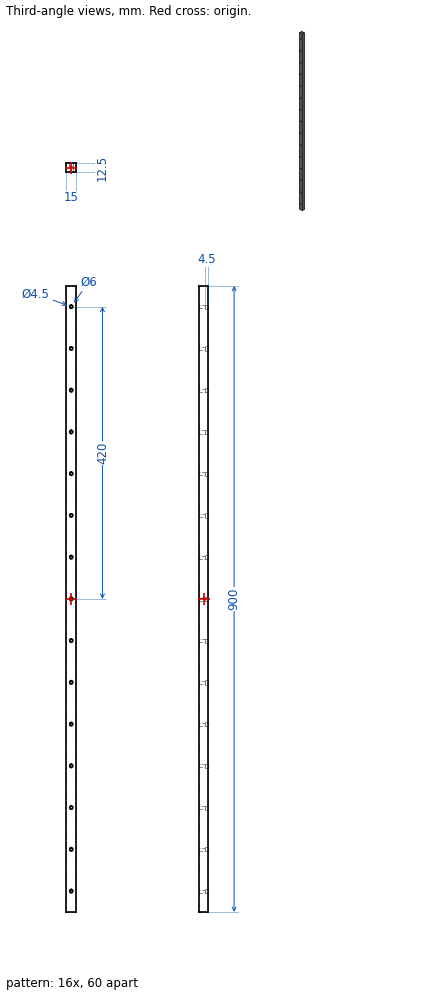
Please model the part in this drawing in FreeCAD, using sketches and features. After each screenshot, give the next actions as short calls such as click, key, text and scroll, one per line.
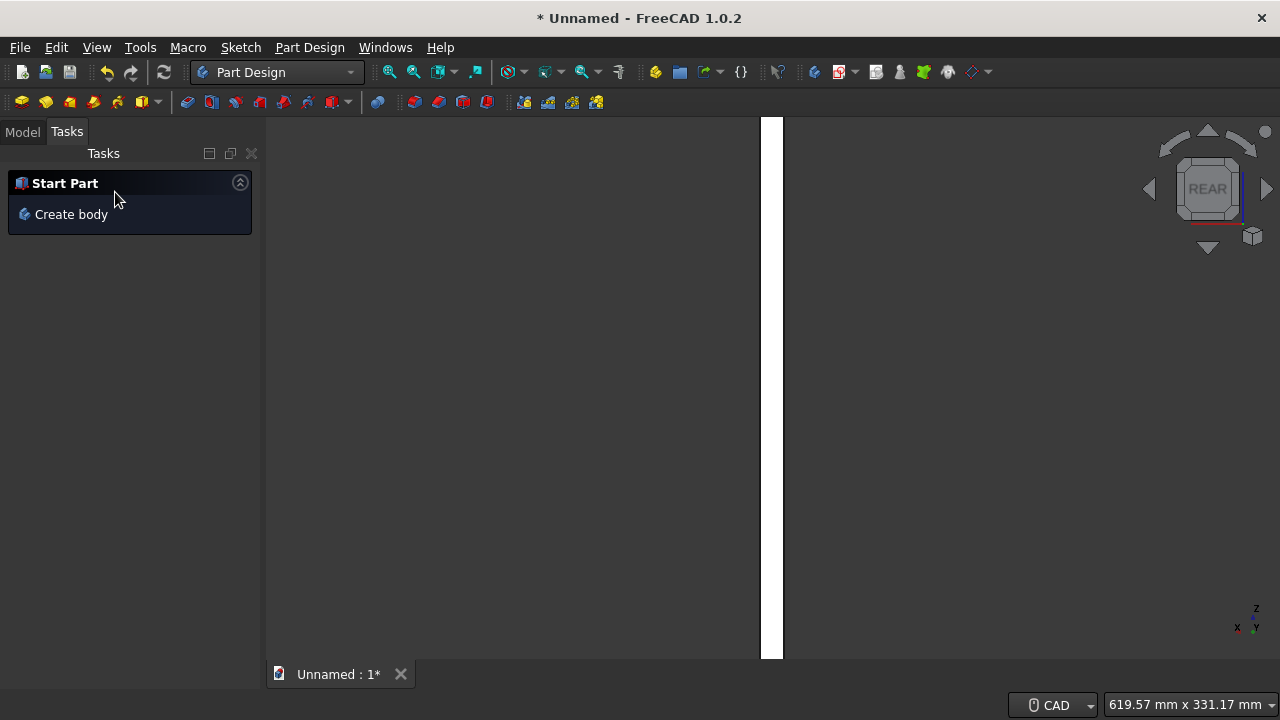
click(390, 72)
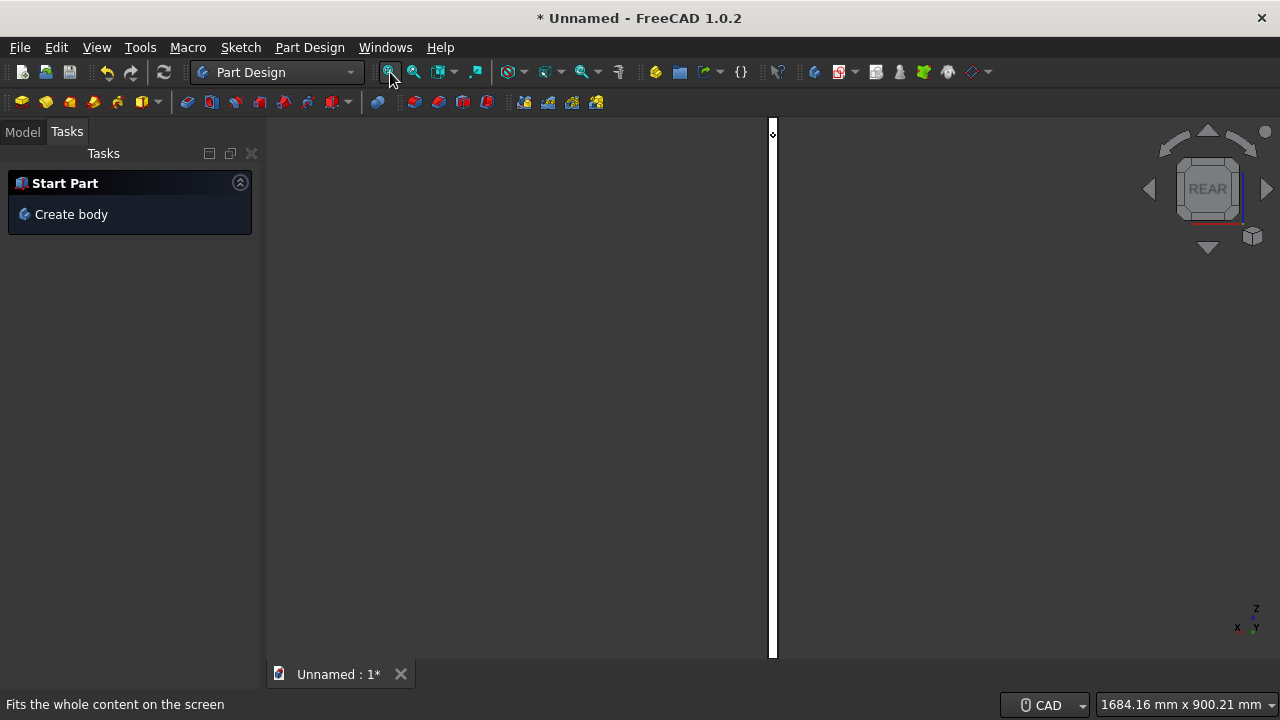
scroll(773, 155, up, 5)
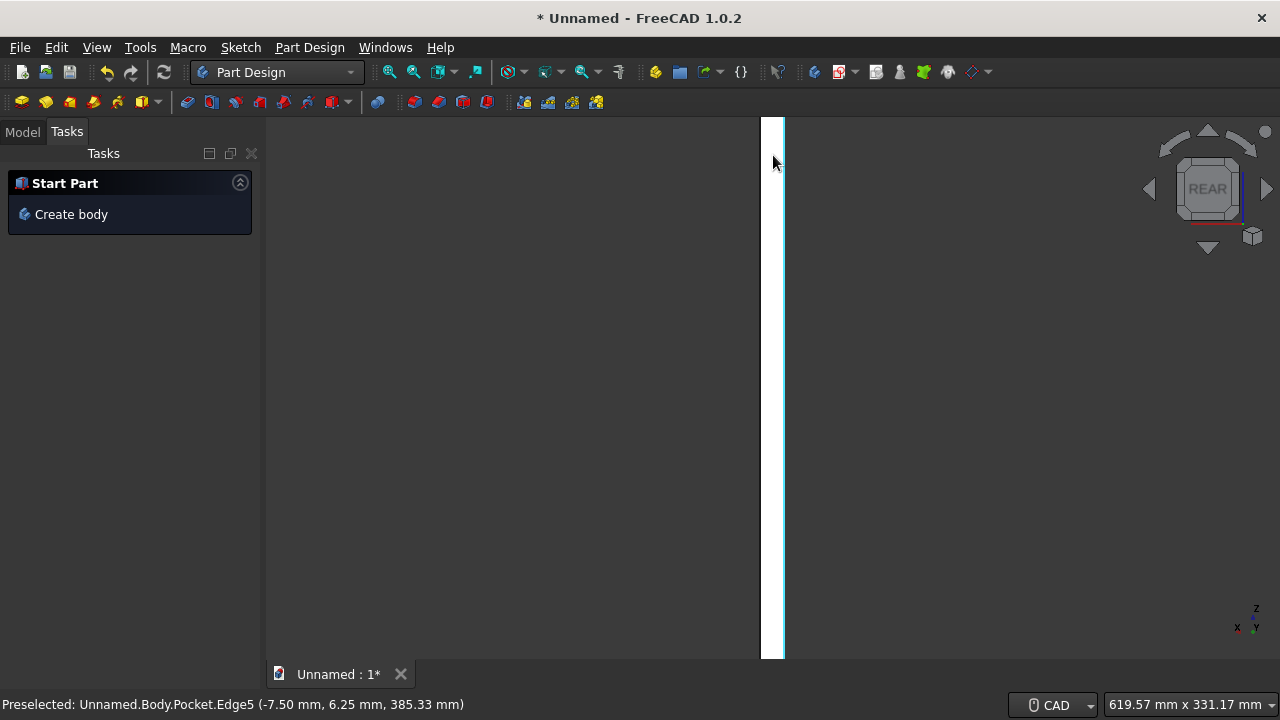
click(772, 156)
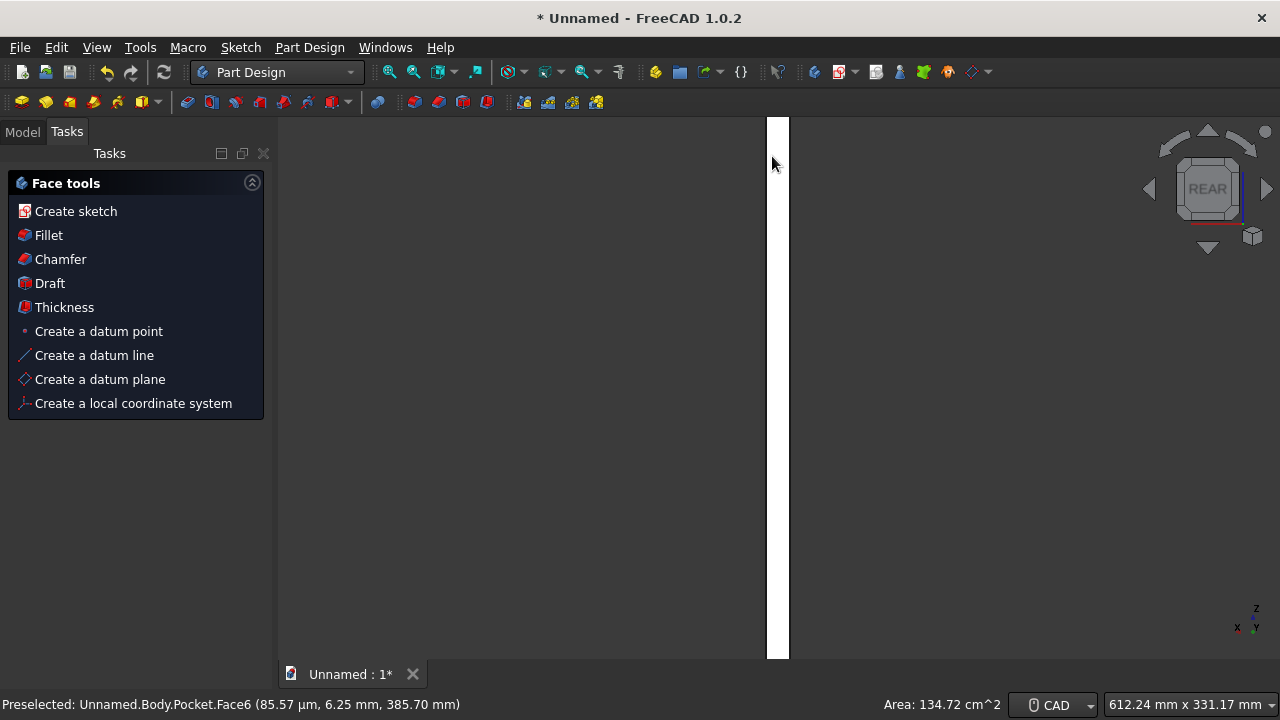
click(840, 72)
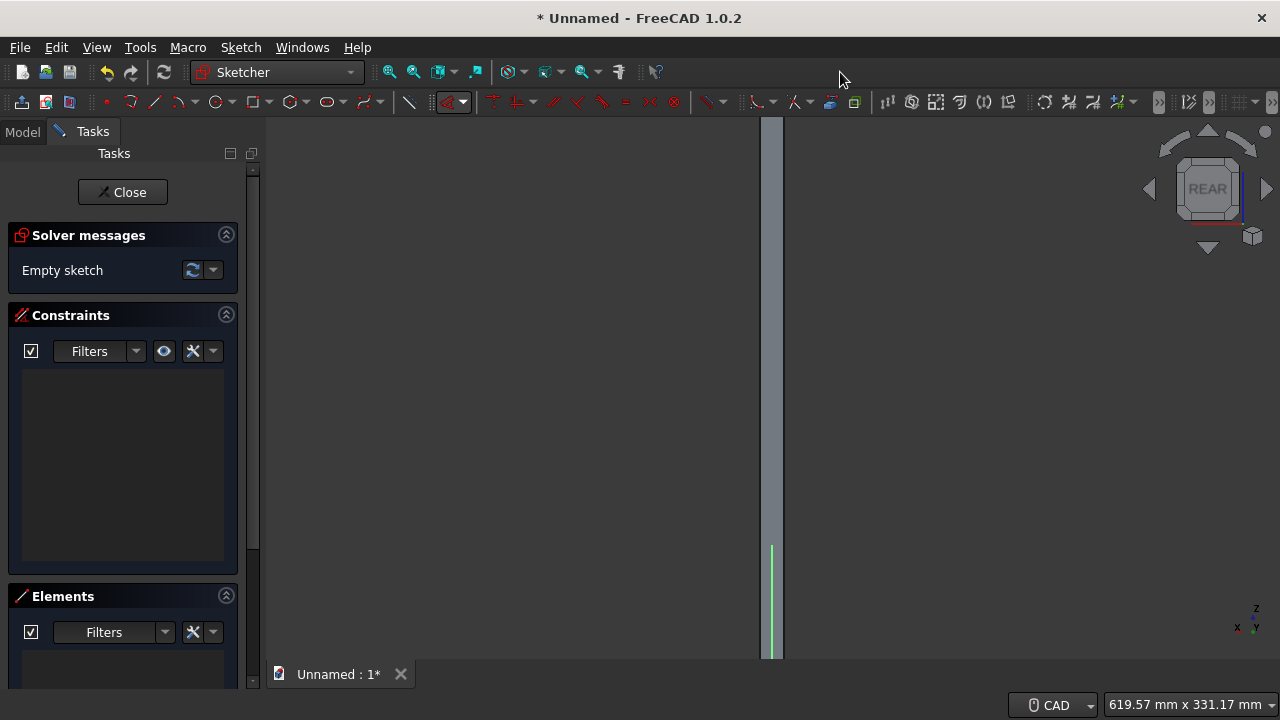
scroll(704, 388, down, 5)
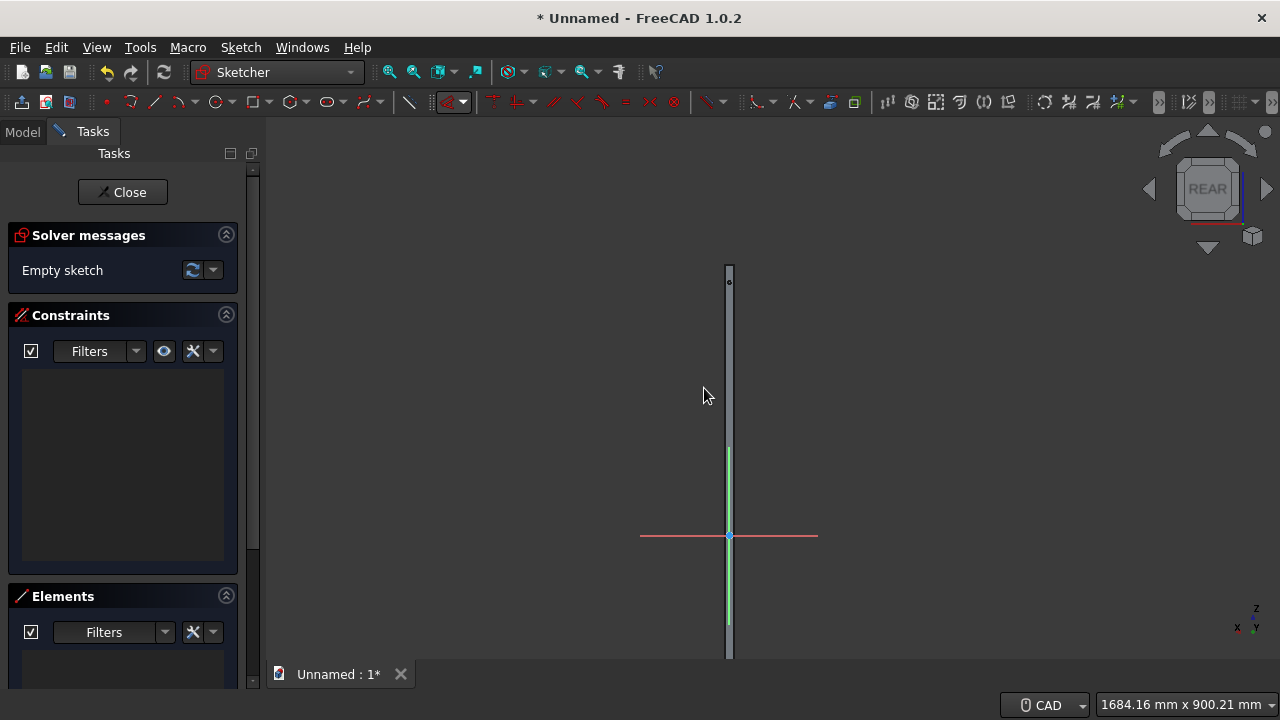
scroll(731, 277, up, 15)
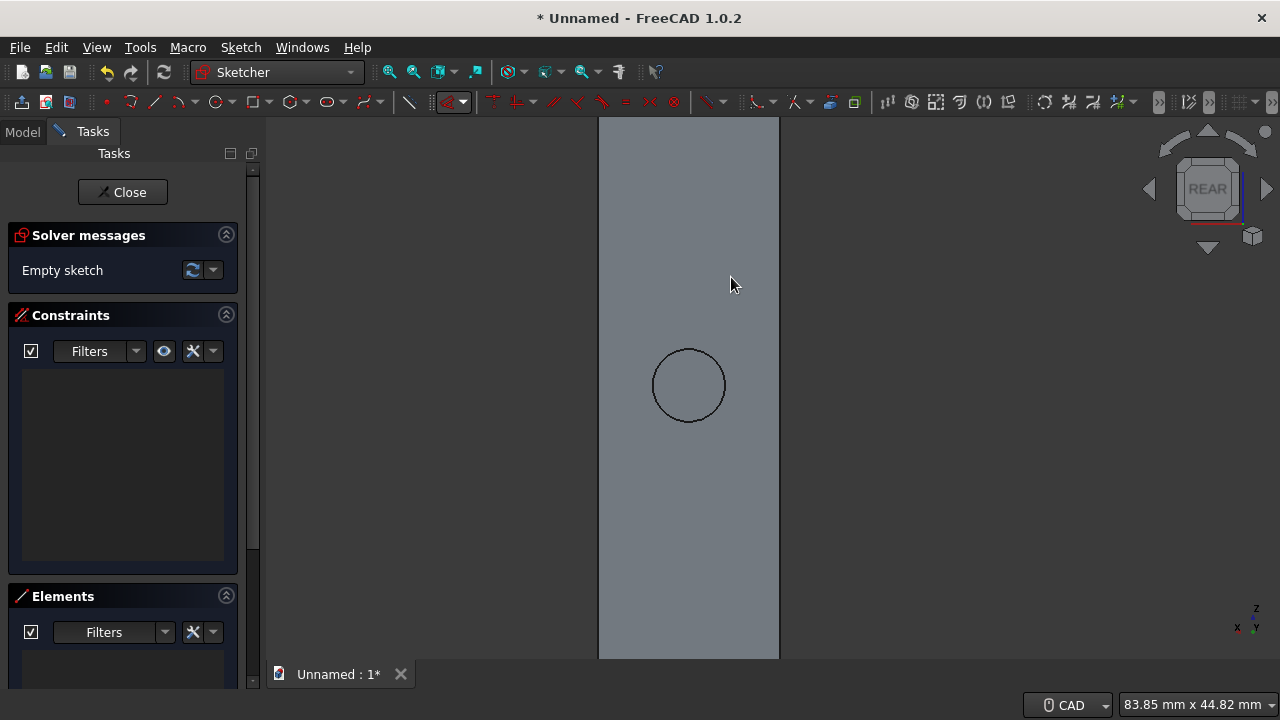
scroll(686, 385, up, 9)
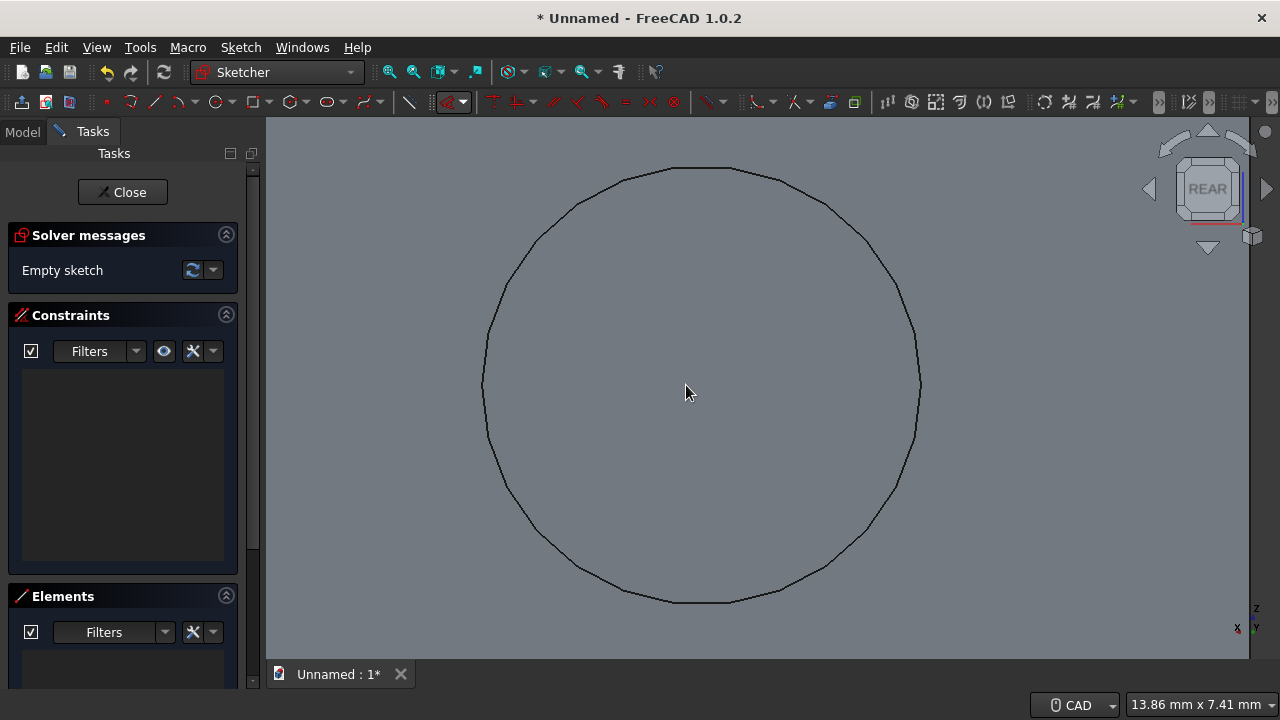
click(216, 102)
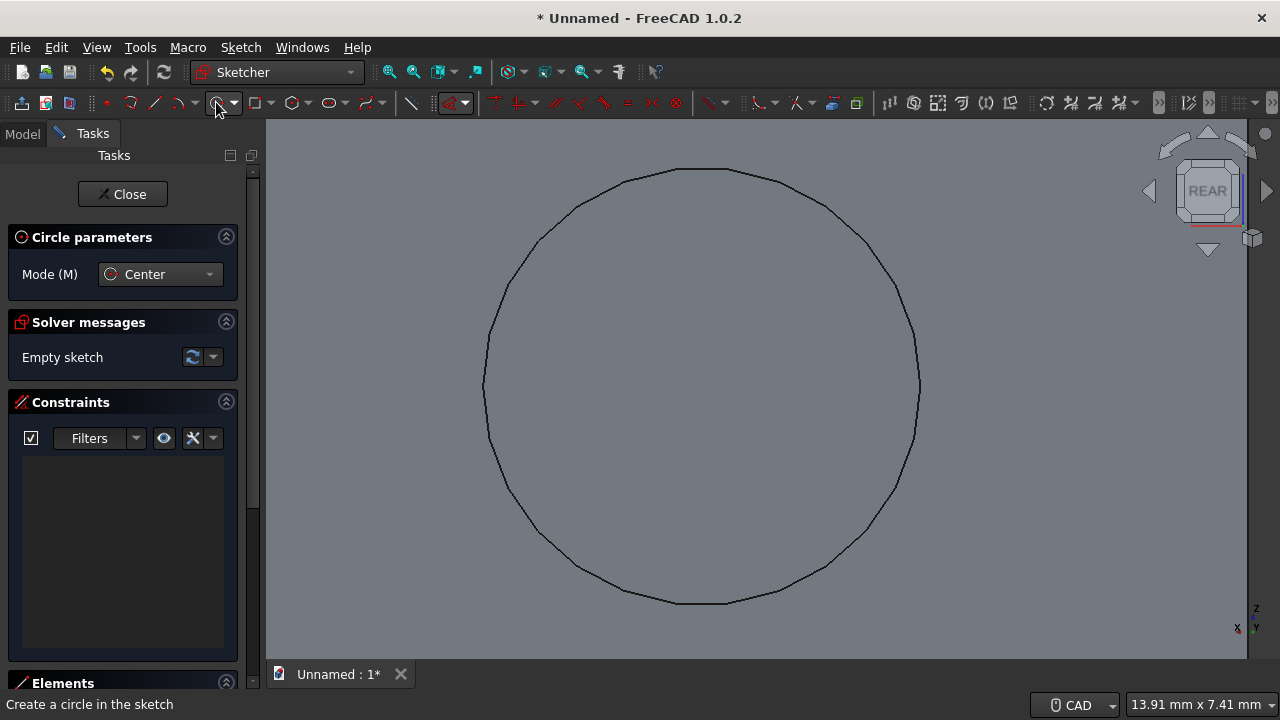
click(702, 386)
move(818, 271)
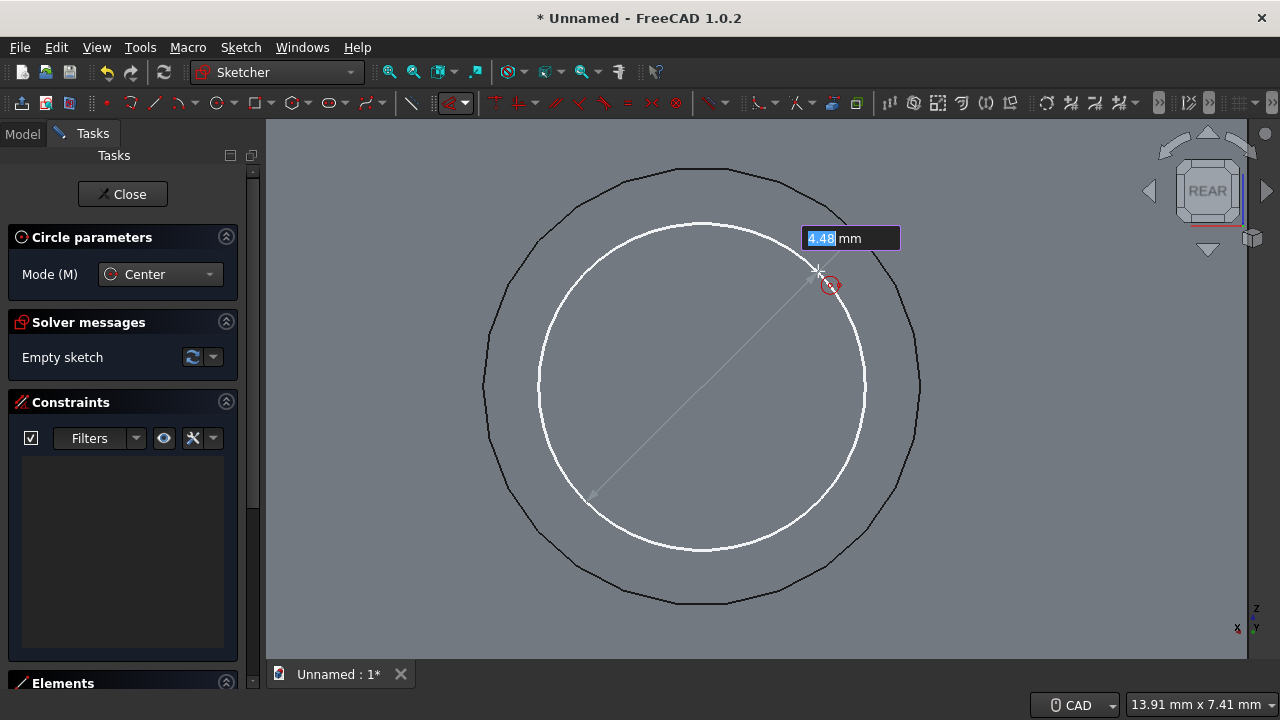
text(4.5)
key(Return)
key(Escape)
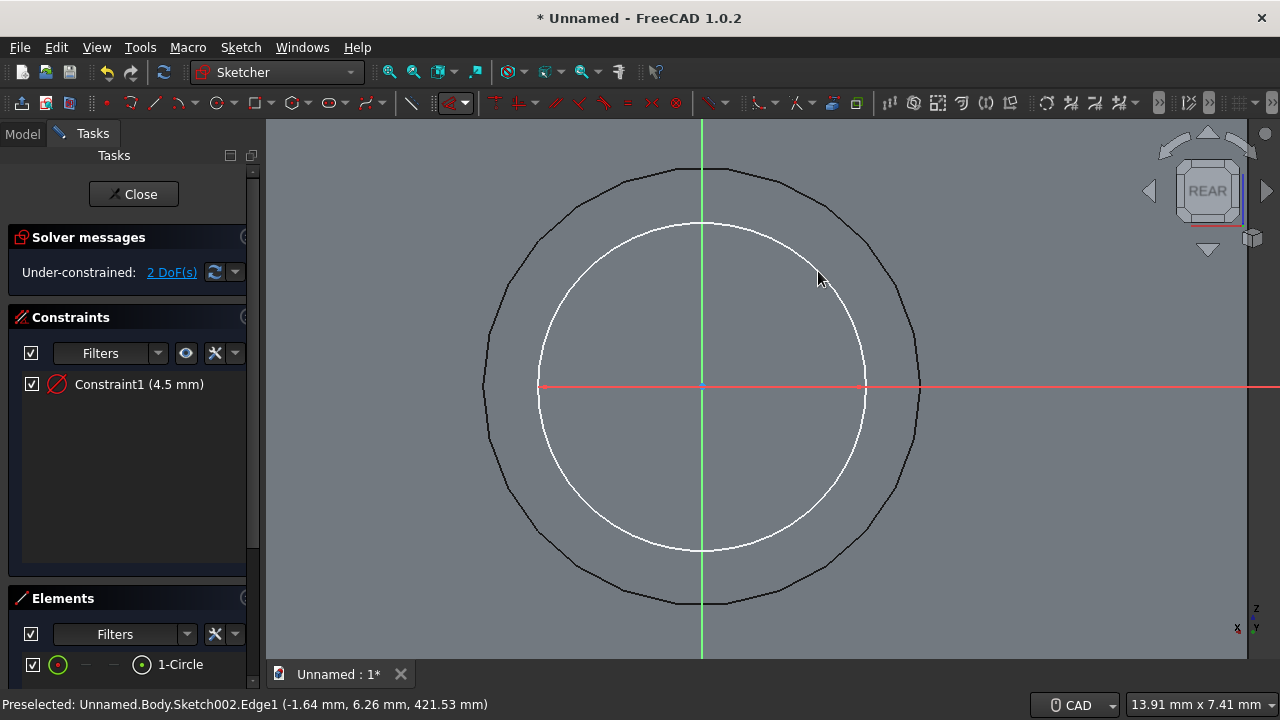
click(702, 387)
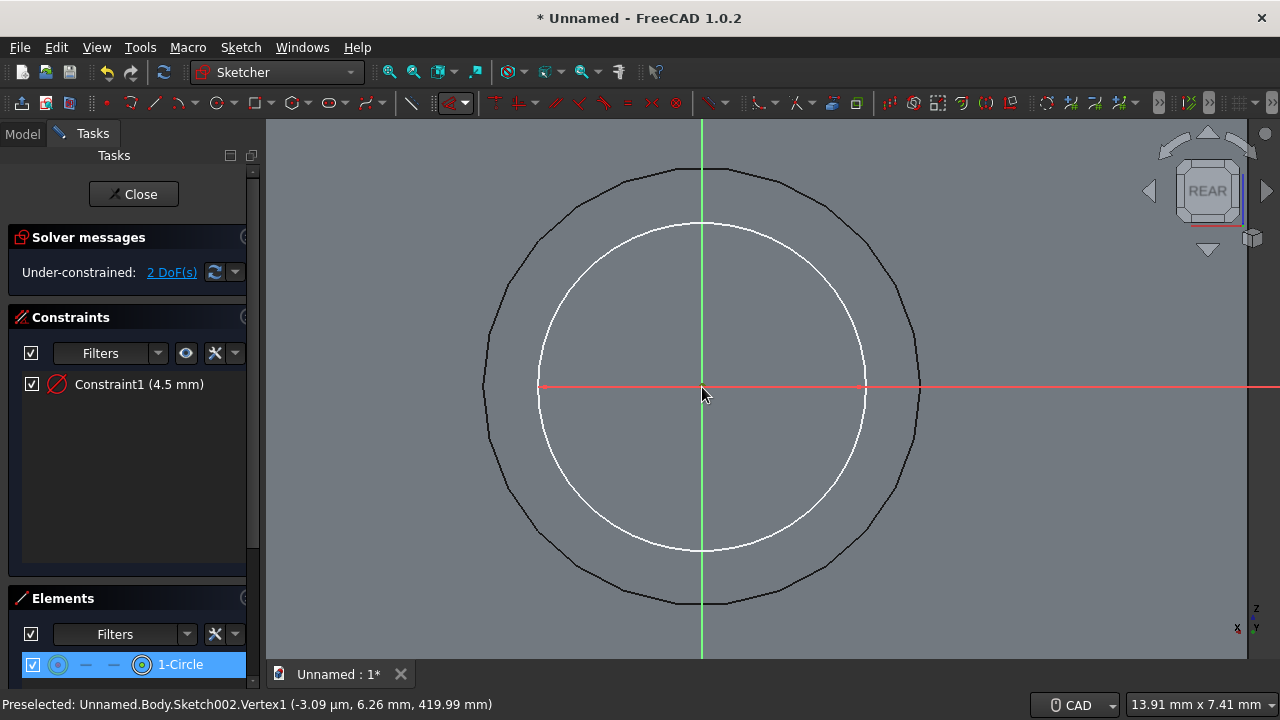
click(702, 596)